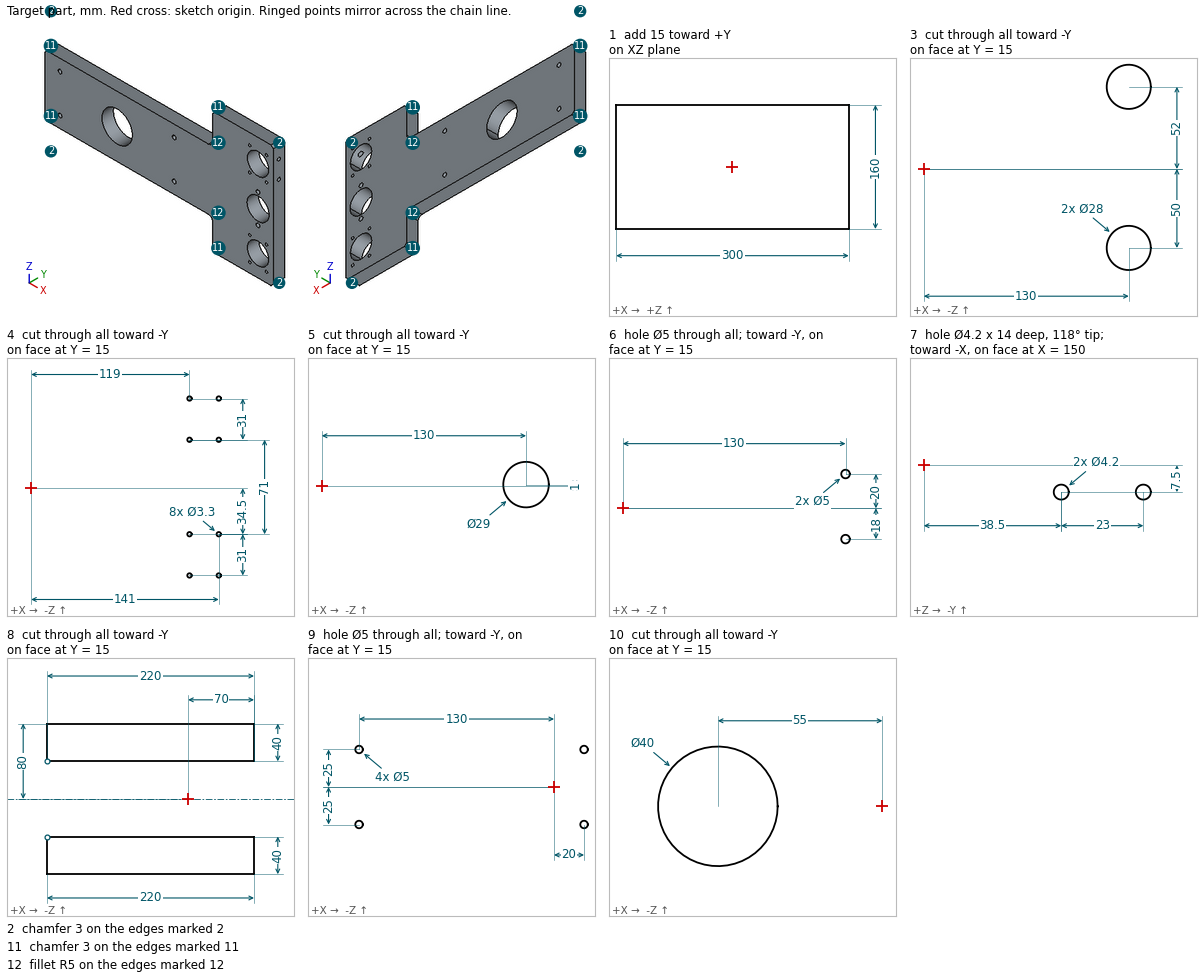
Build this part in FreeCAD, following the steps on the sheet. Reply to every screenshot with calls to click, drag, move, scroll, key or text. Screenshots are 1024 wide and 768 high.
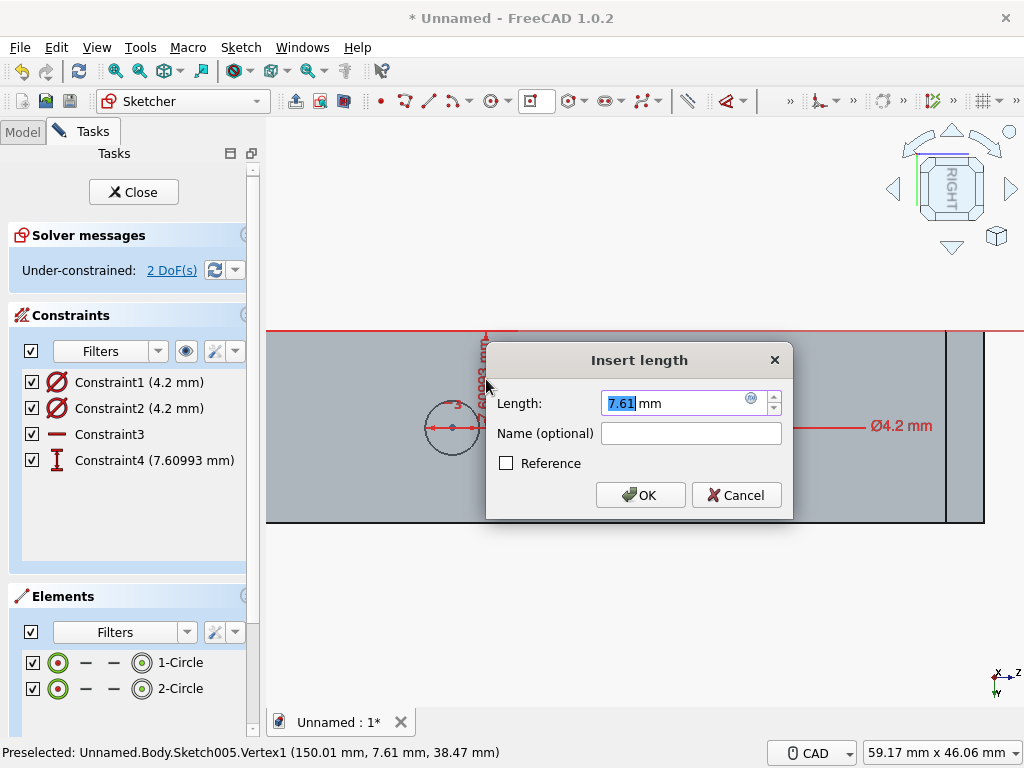
text(7.5)
key(Return)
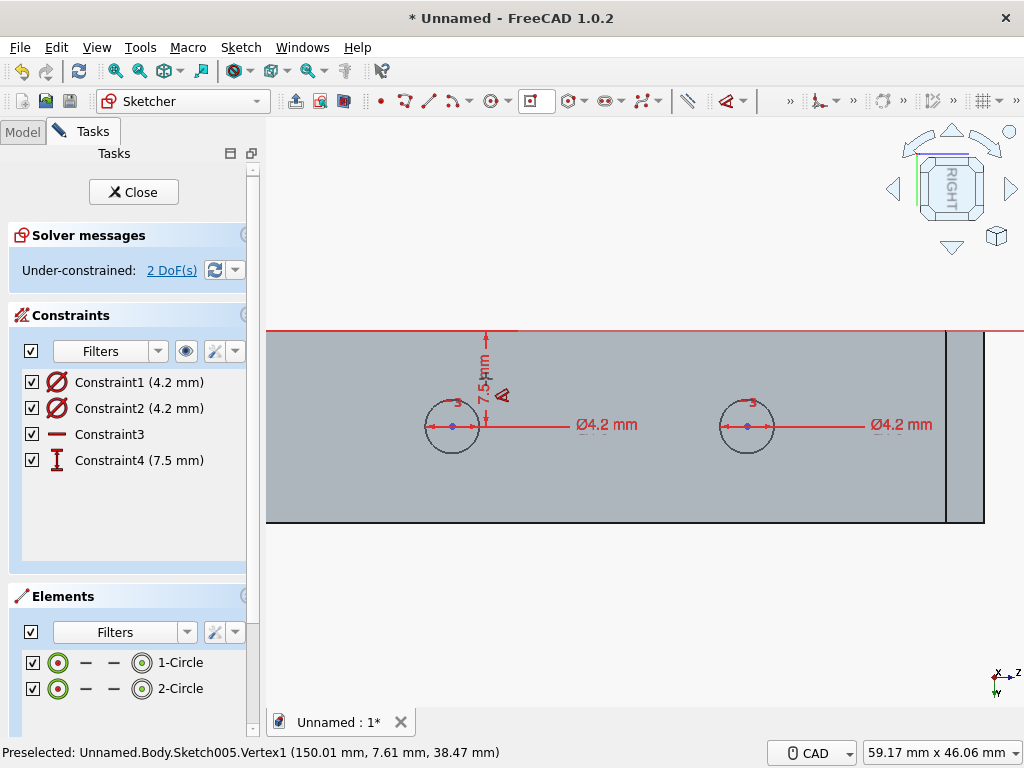
click(452, 427)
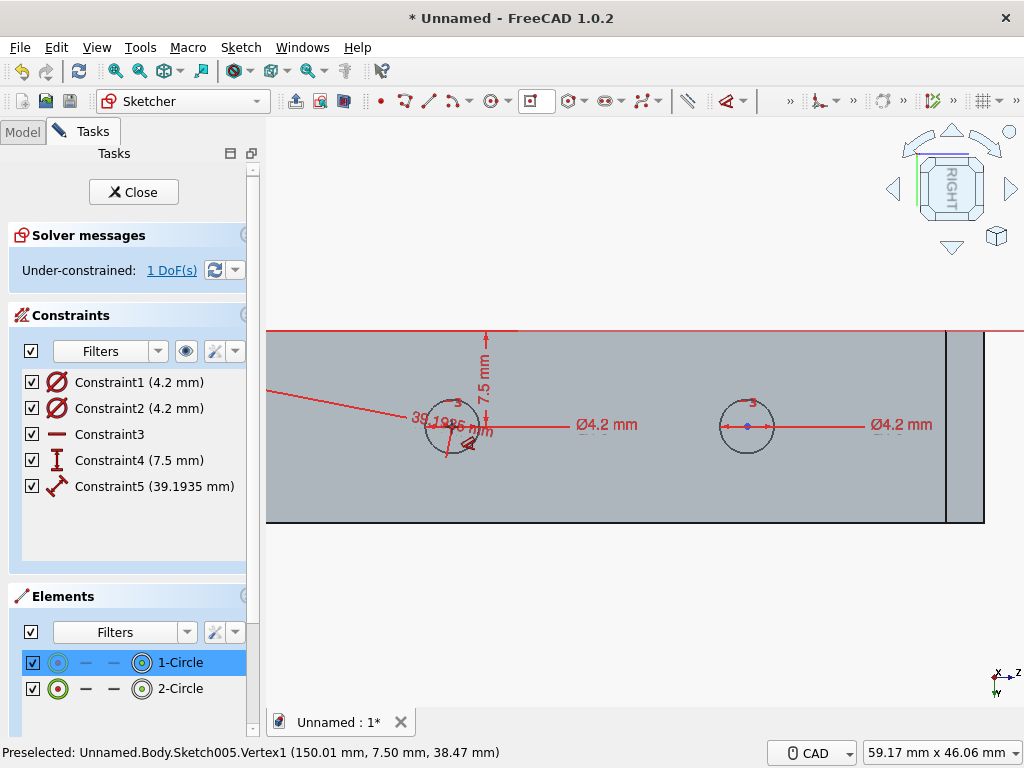
click(747, 427)
click(600, 461)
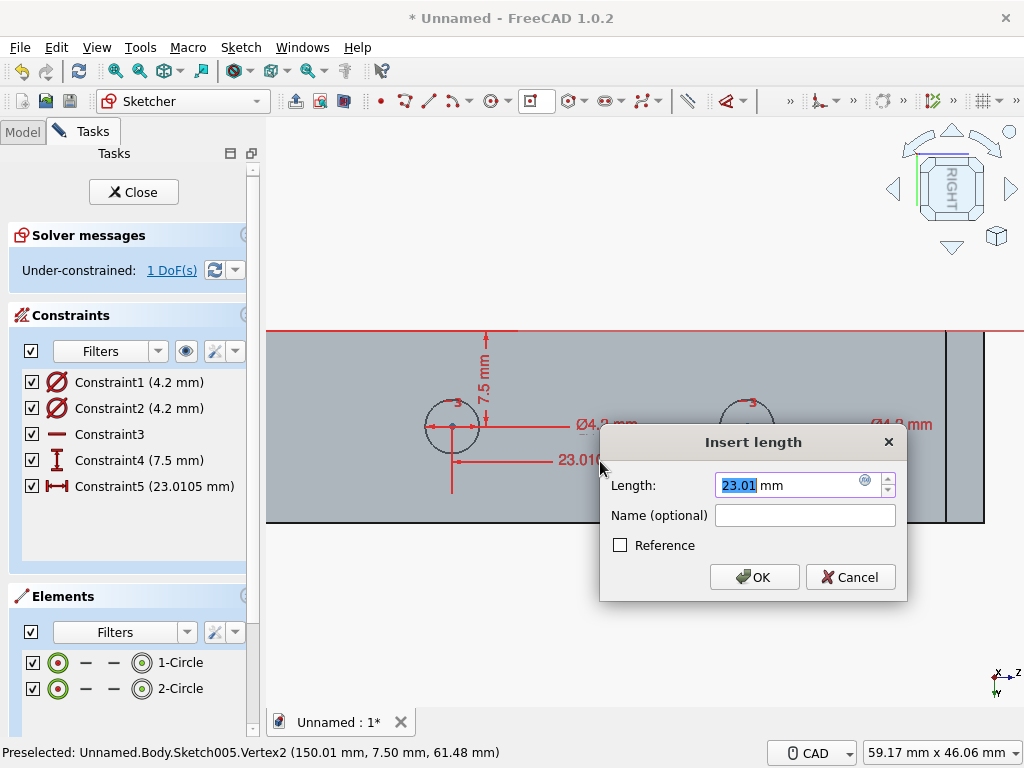
text(23)
key(Return)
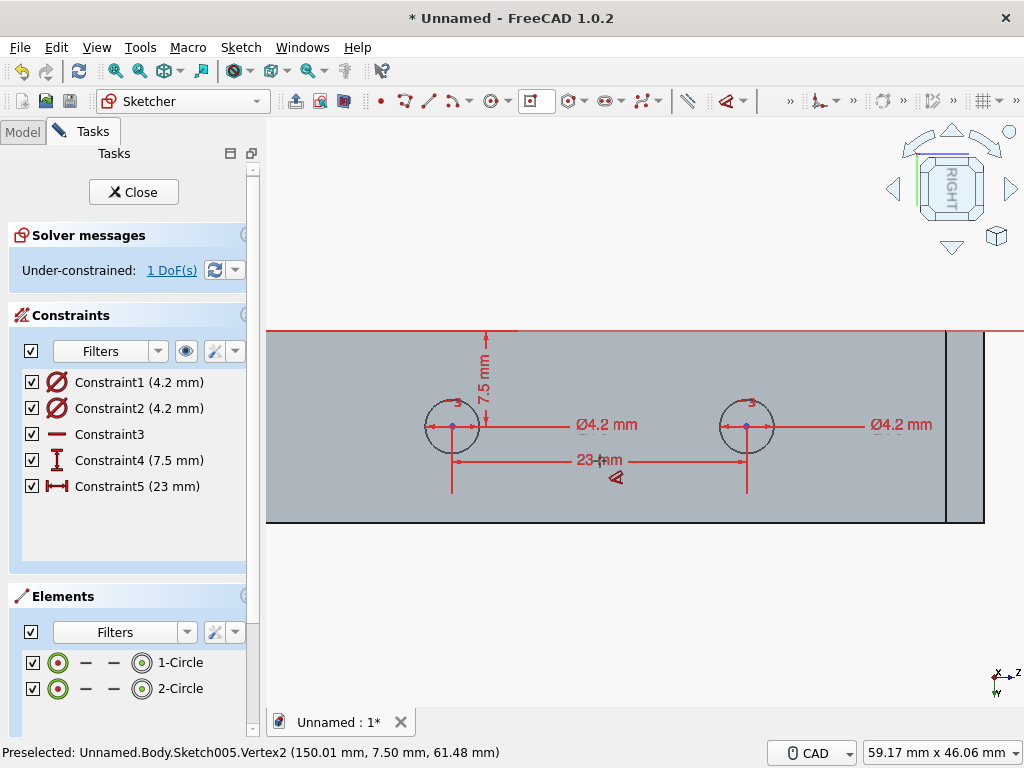
click(452, 427)
click(373, 297)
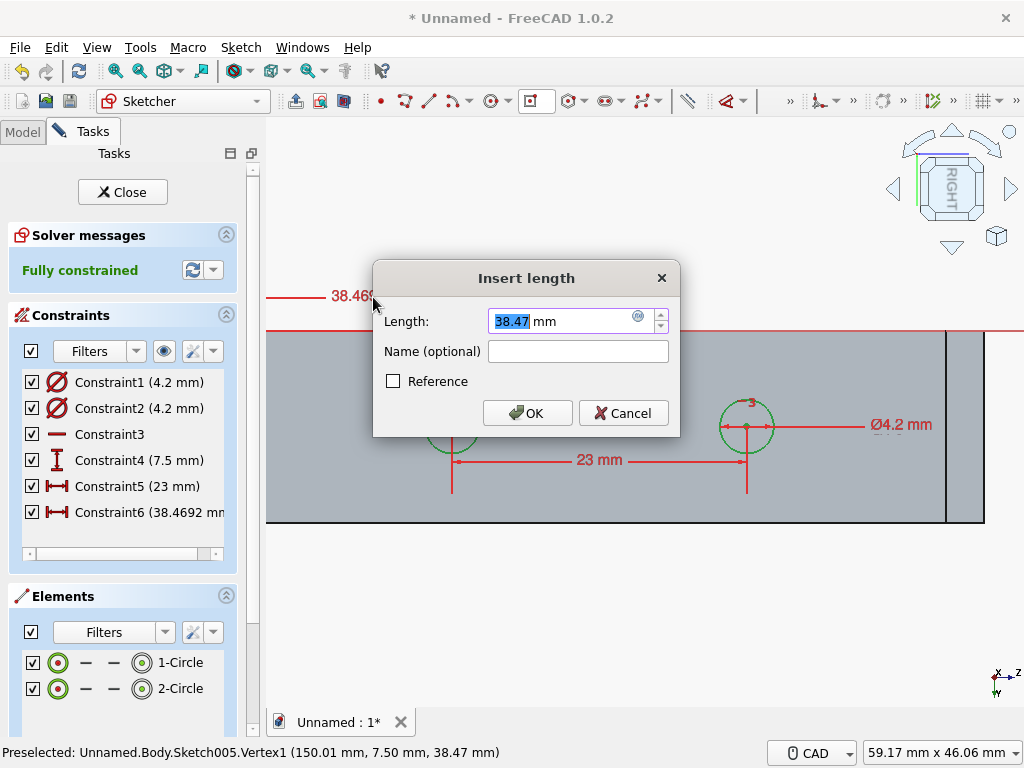
text(38.5)
key(Return)
key(Escape)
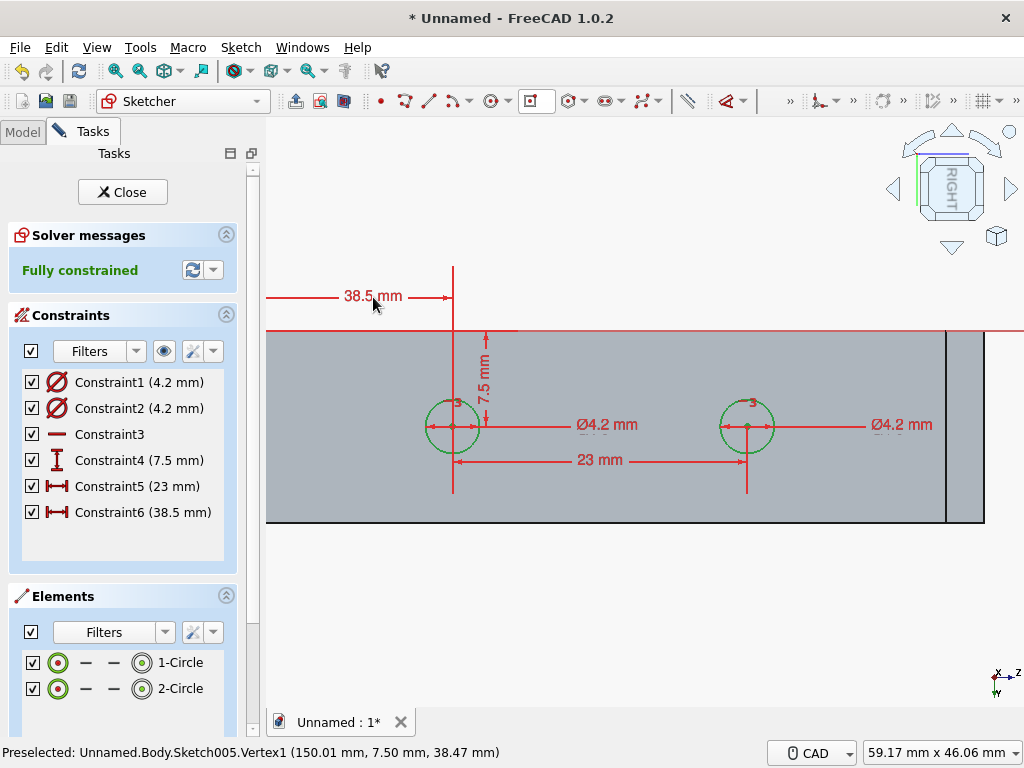
click(123, 192)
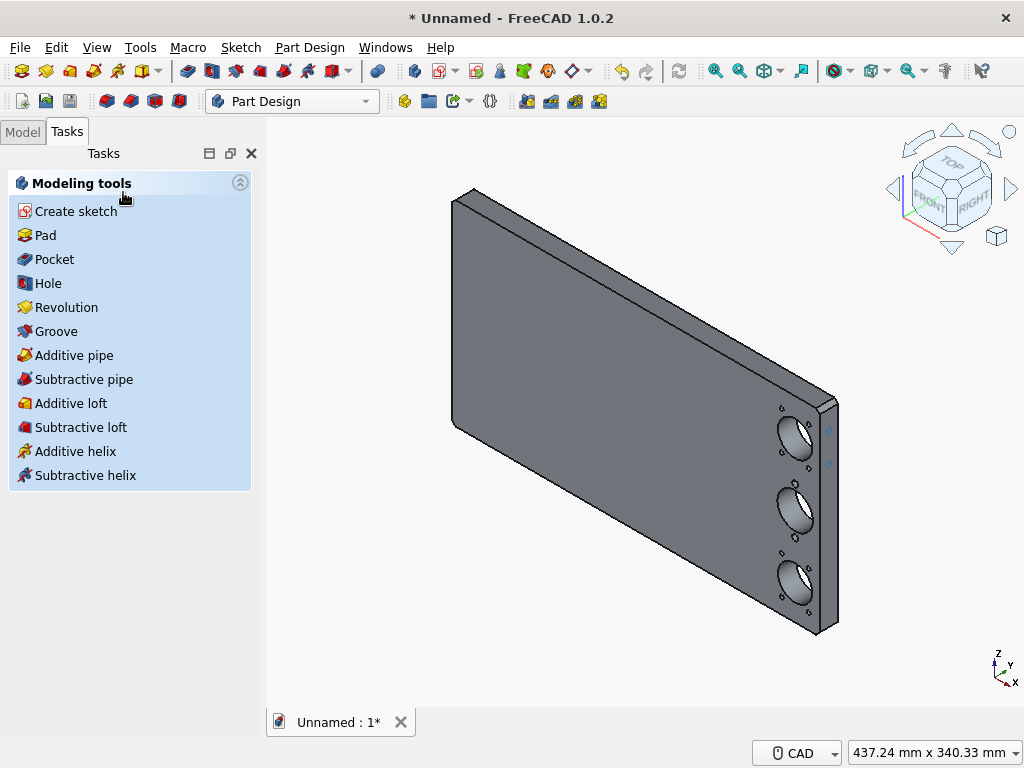
click(212, 72)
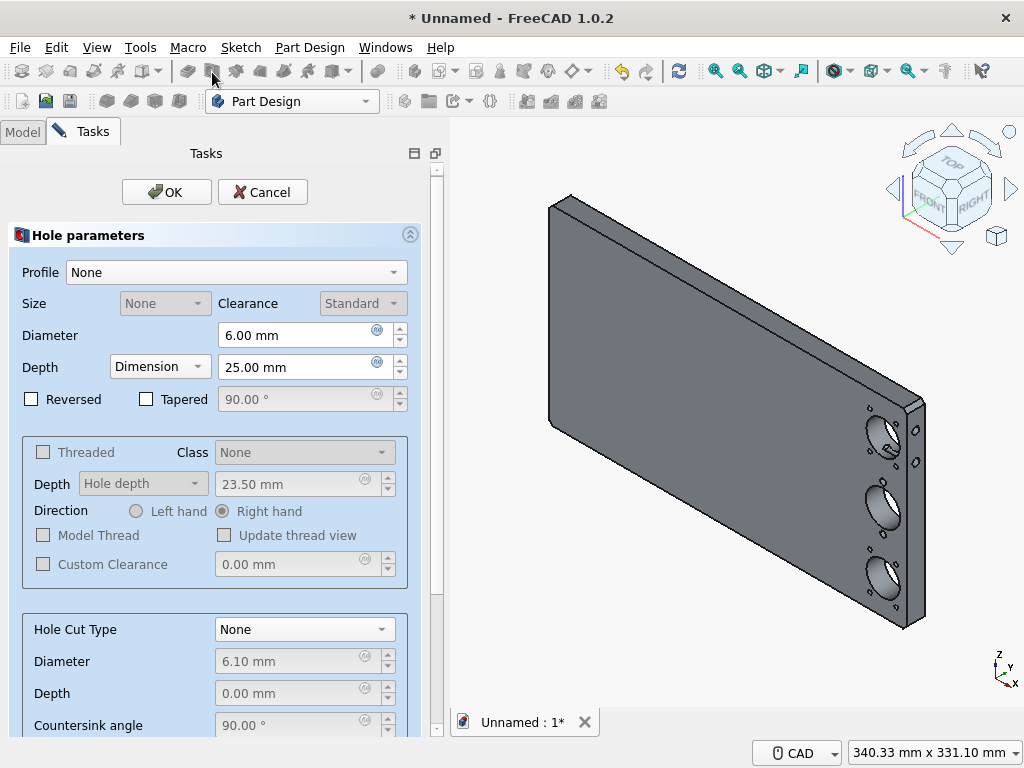
triple_click(305, 335)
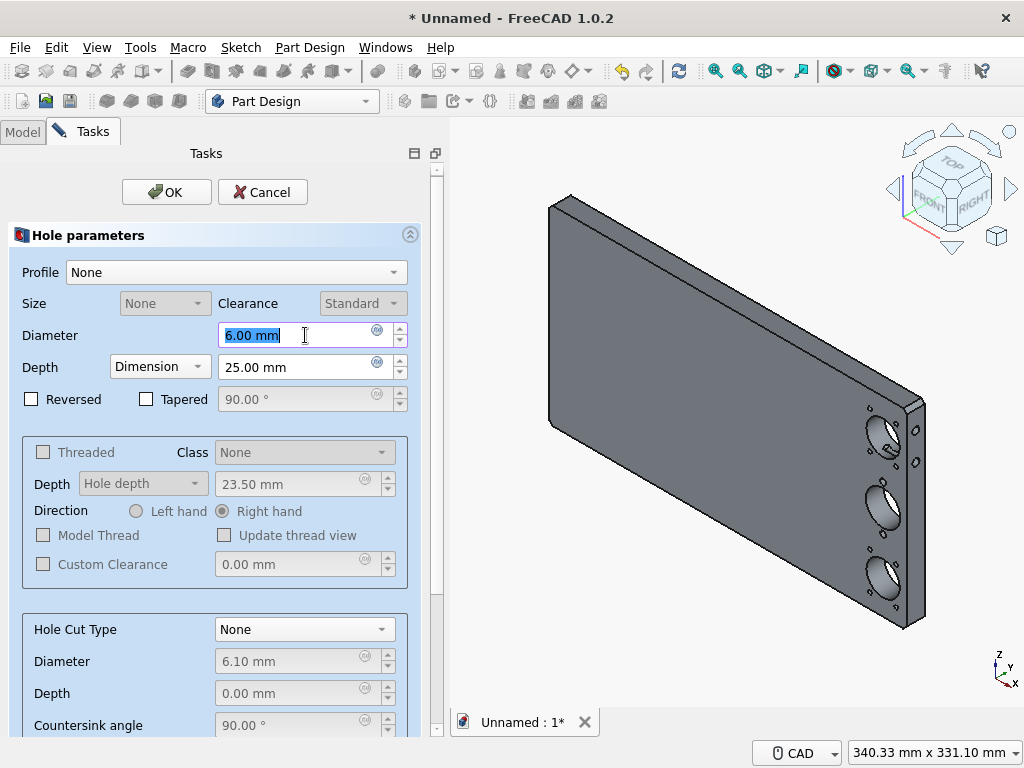
text(4.2)
key(Tab)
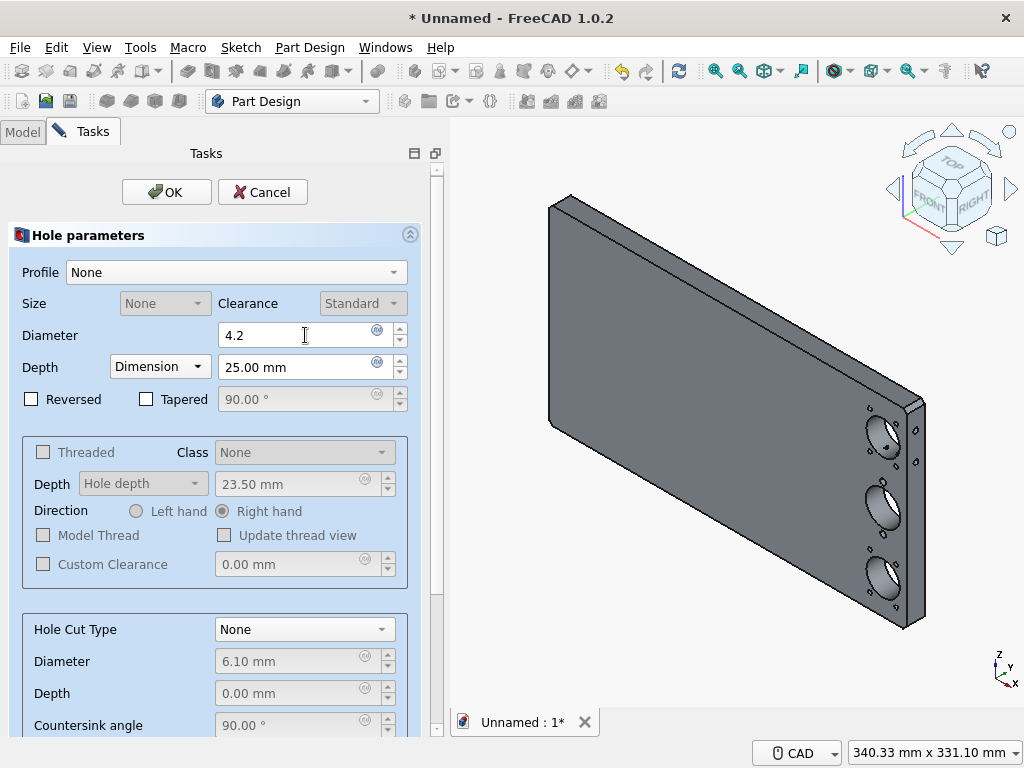
triple_click(305, 367)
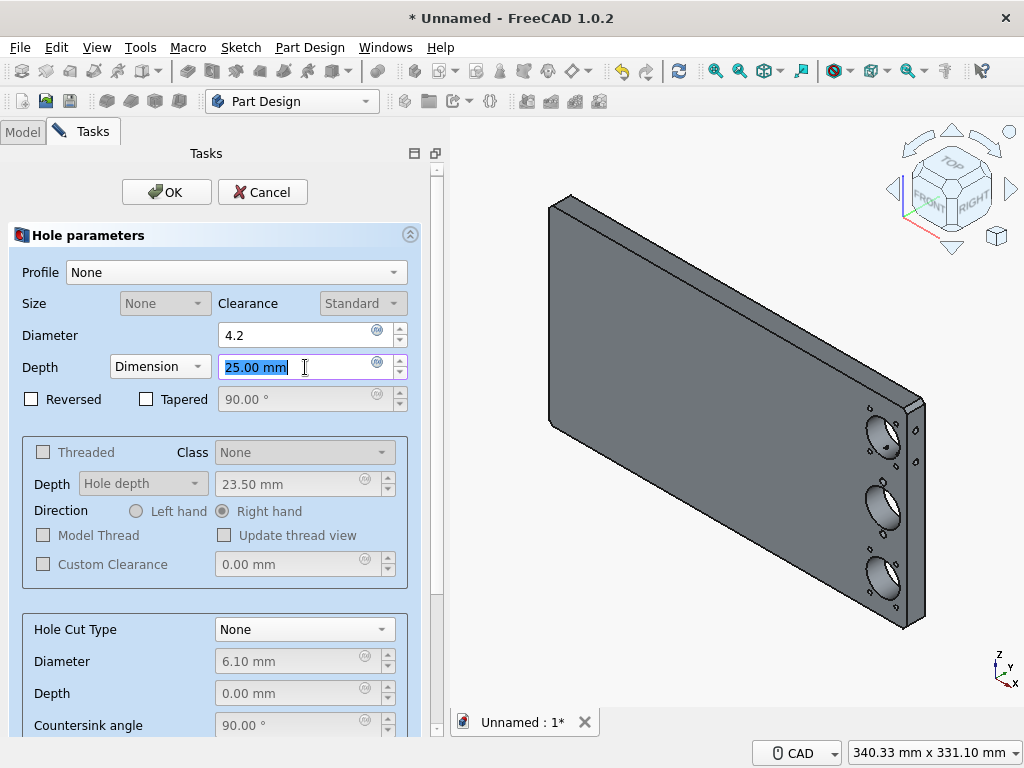
text(14)
key(Tab)